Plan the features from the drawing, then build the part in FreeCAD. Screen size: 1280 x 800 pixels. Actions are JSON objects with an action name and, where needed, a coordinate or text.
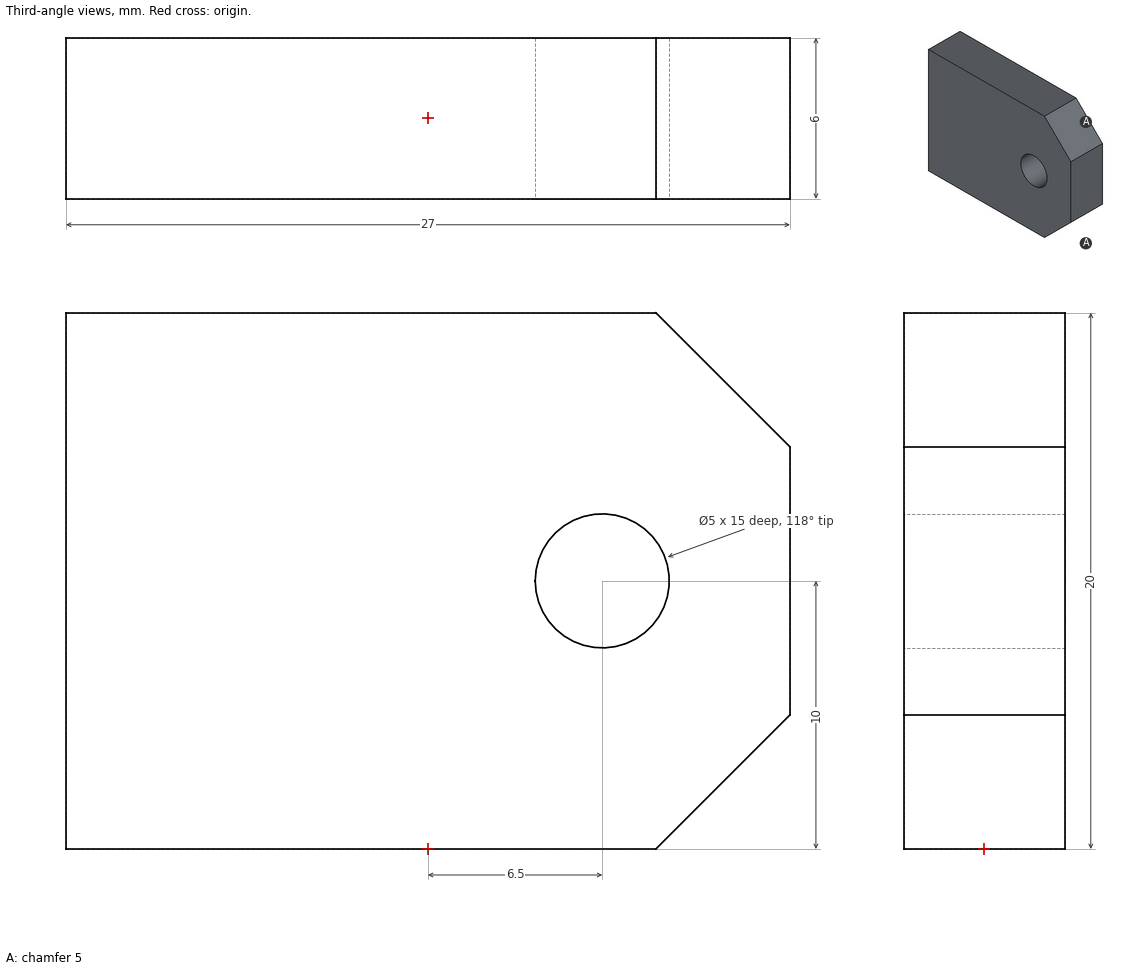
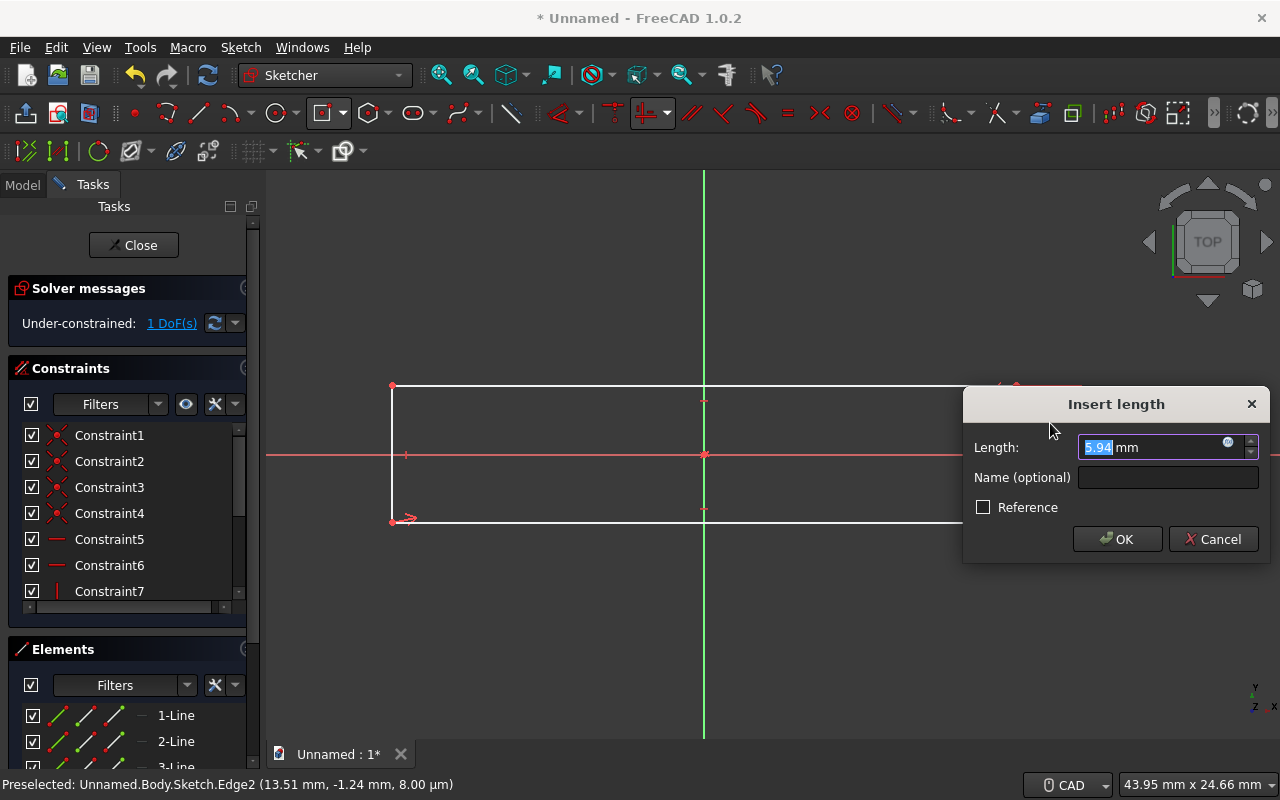
{"action": "type", "text": "6"}
{"action": "key", "text": "Return"}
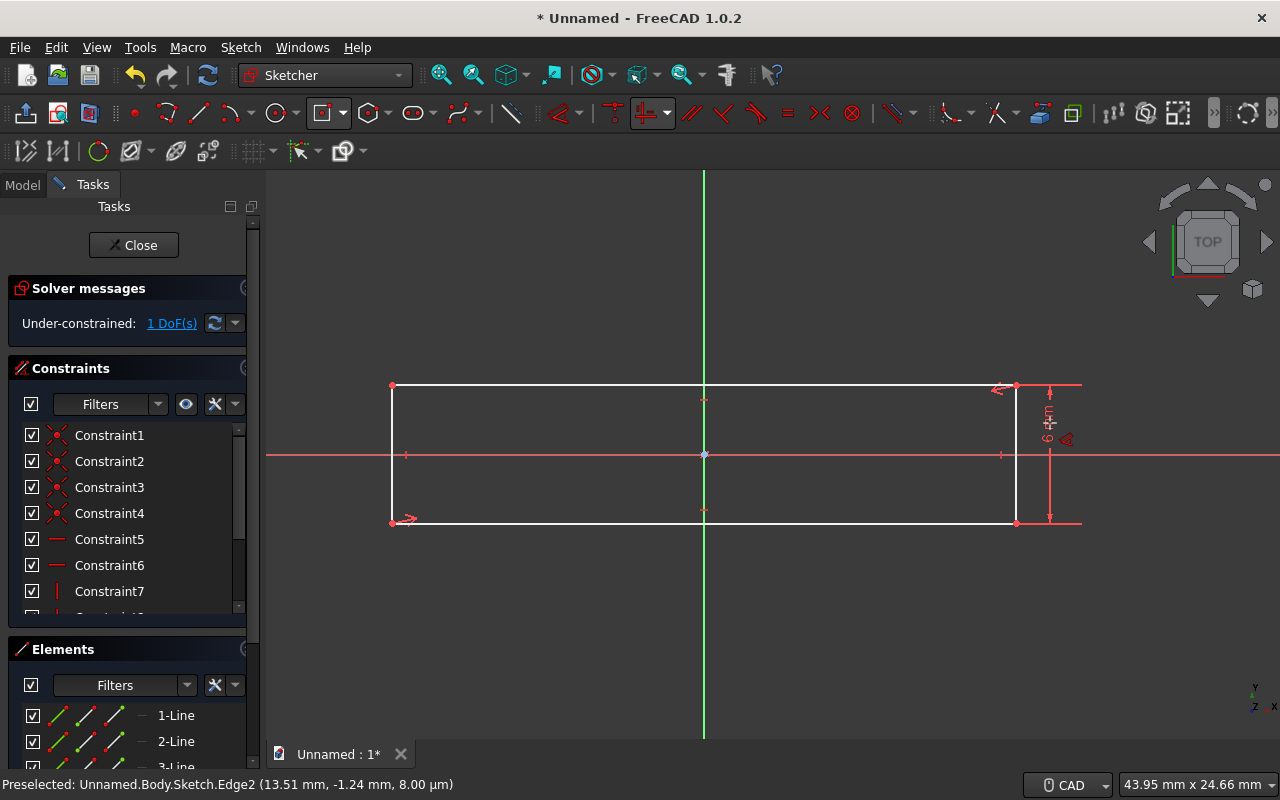
{"action": "left_click", "coordinate": [579, 524]}
{"action": "left_click", "coordinate": [561, 558]}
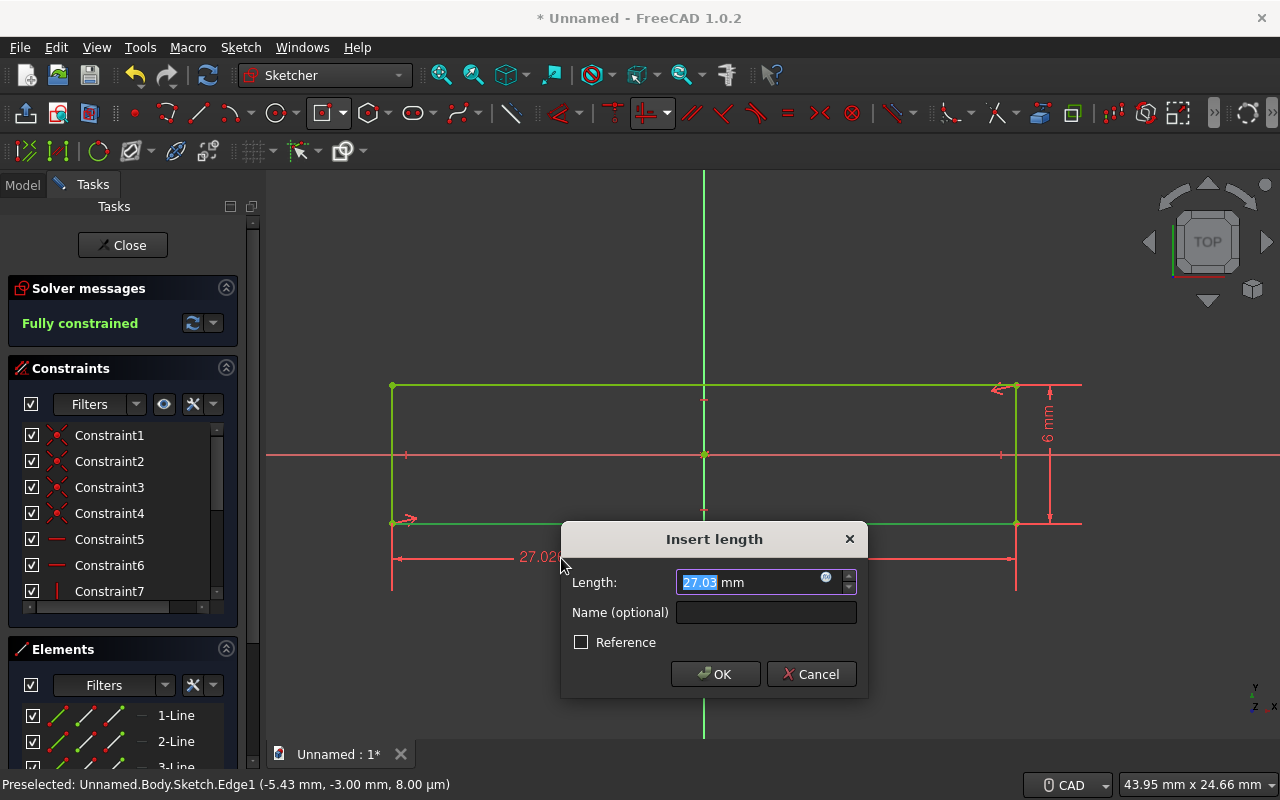
{"action": "type", "text": "27"}
{"action": "key", "text": "Return"}
{"action": "key", "text": "Escape"}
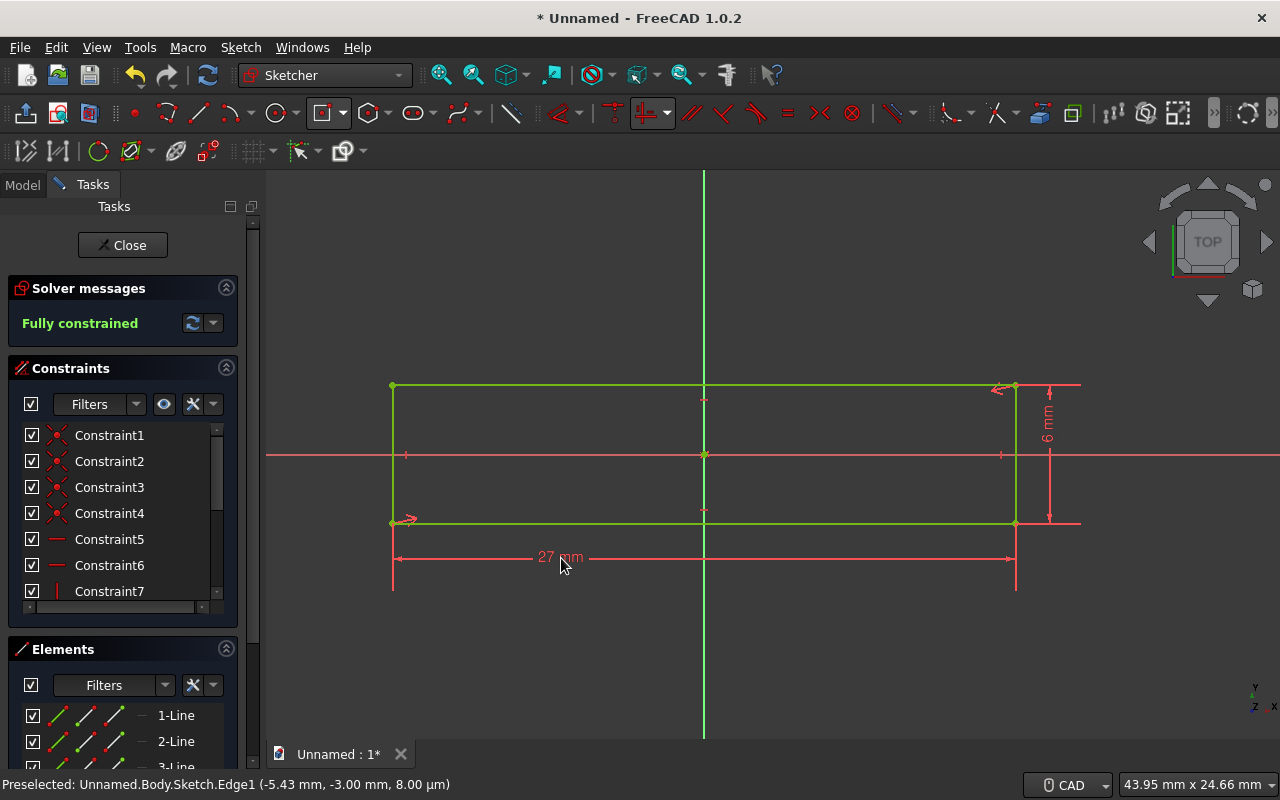
{"action": "left_click", "coordinate": [123, 245]}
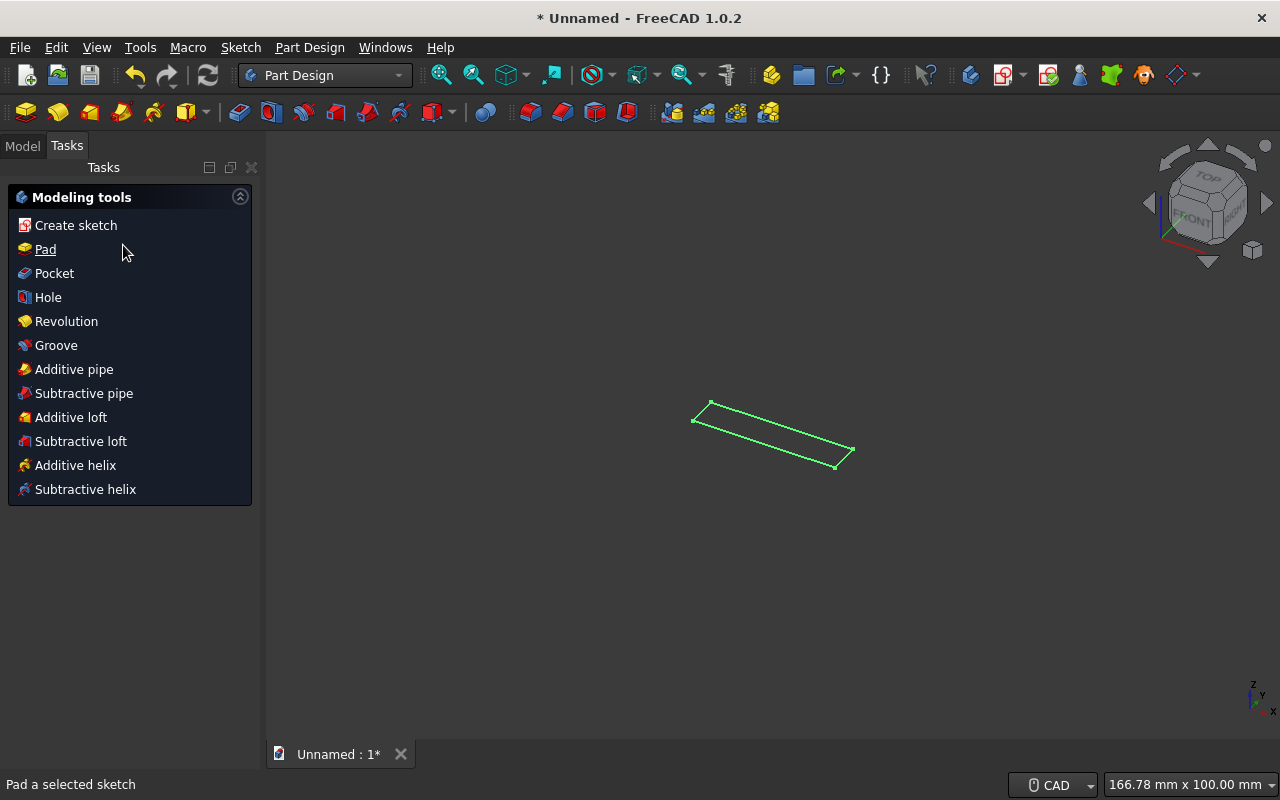
{"action": "left_click", "coordinate": [26, 112]}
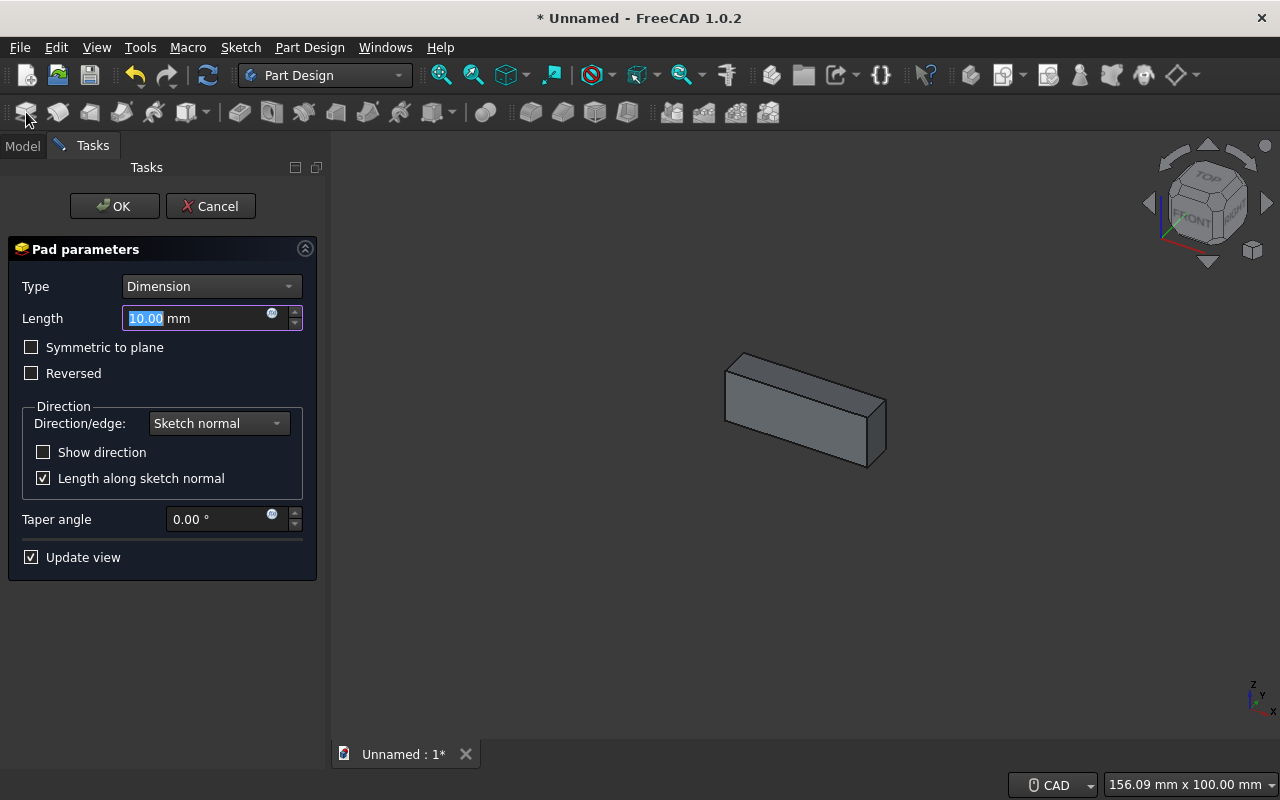
{"action": "type", "text": "20"}
{"action": "key", "text": "Tab"}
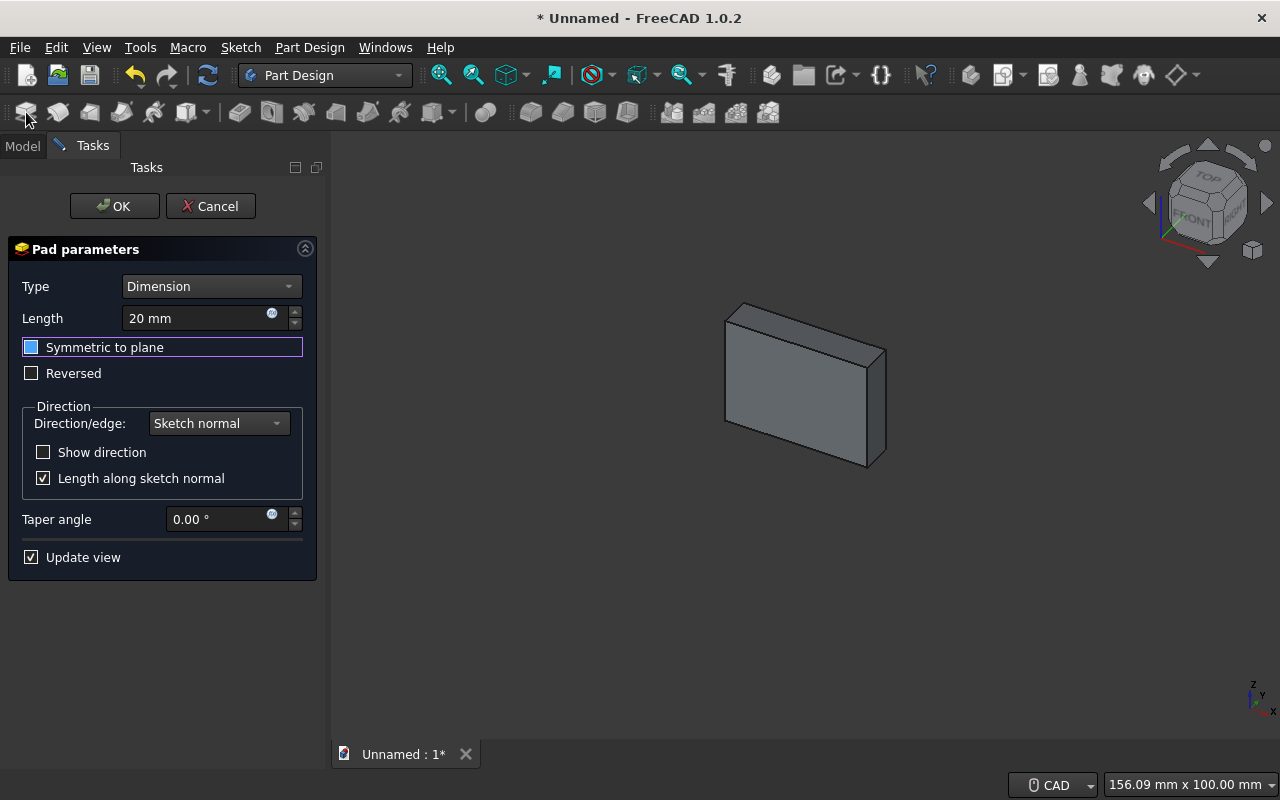
{"action": "left_click", "coordinate": [115, 206]}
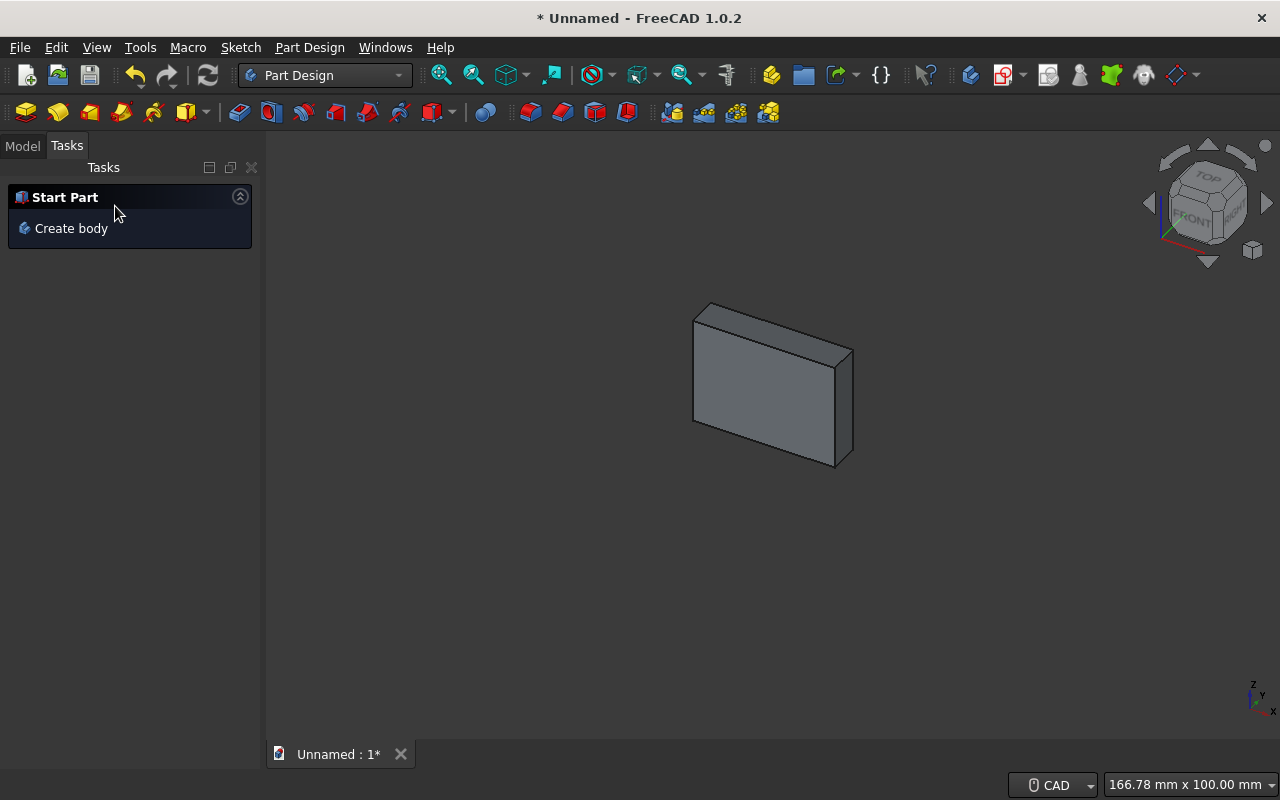
{"action": "left_click", "coordinate": [442, 76]}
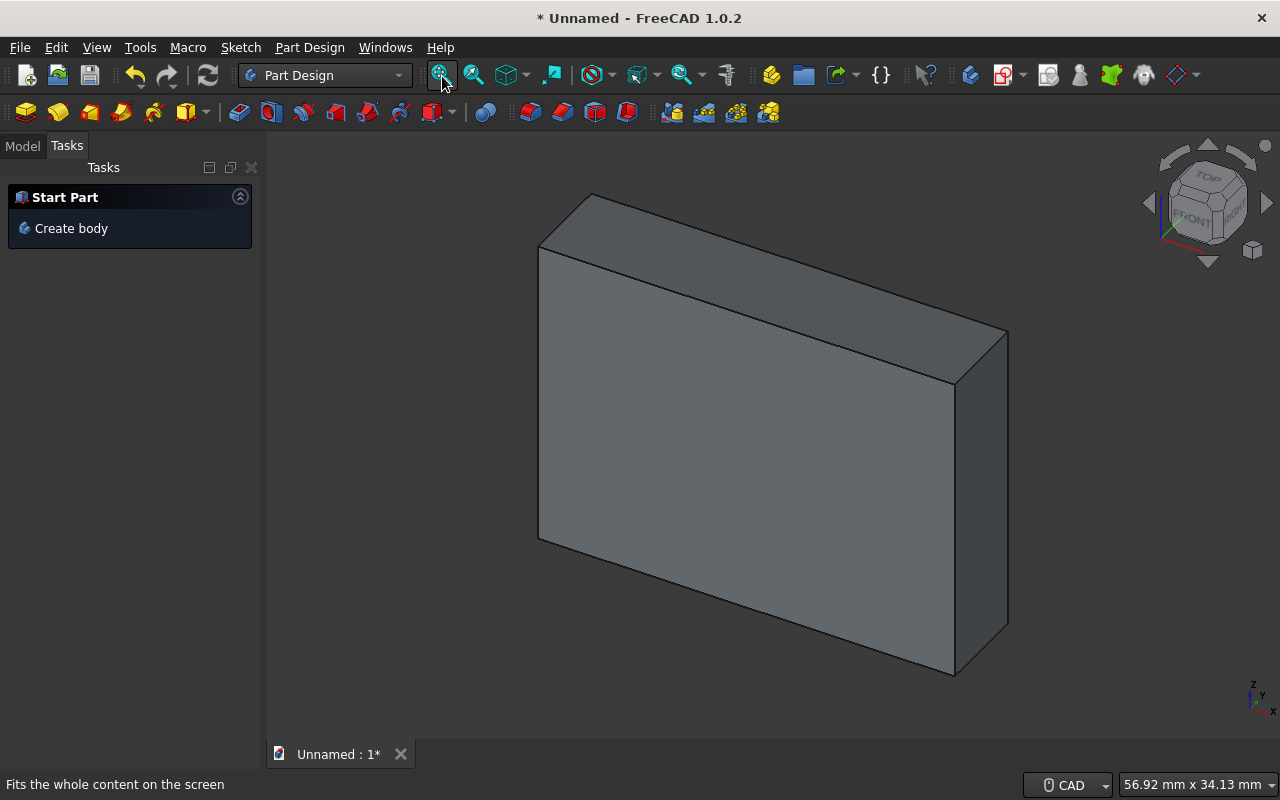
{"action": "key", "text": "4"}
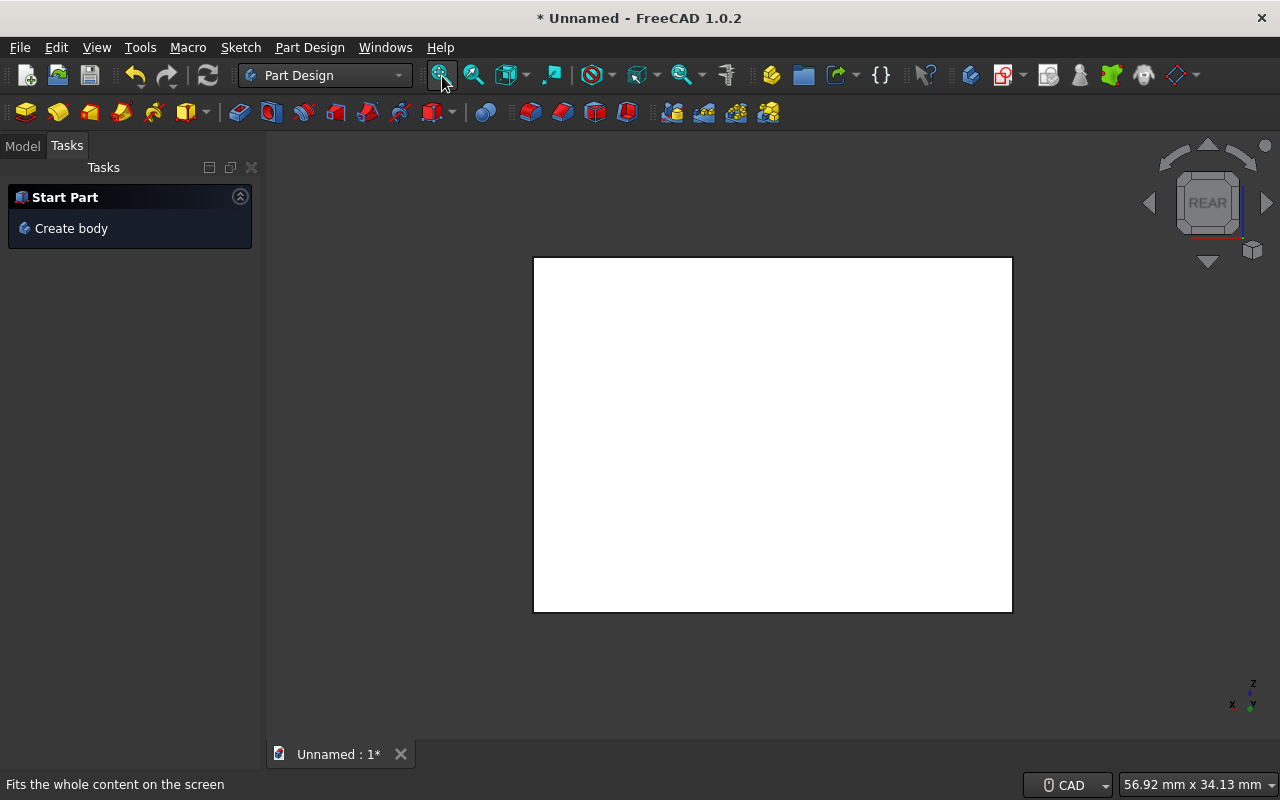
{"action": "left_click", "coordinate": [773, 434]}